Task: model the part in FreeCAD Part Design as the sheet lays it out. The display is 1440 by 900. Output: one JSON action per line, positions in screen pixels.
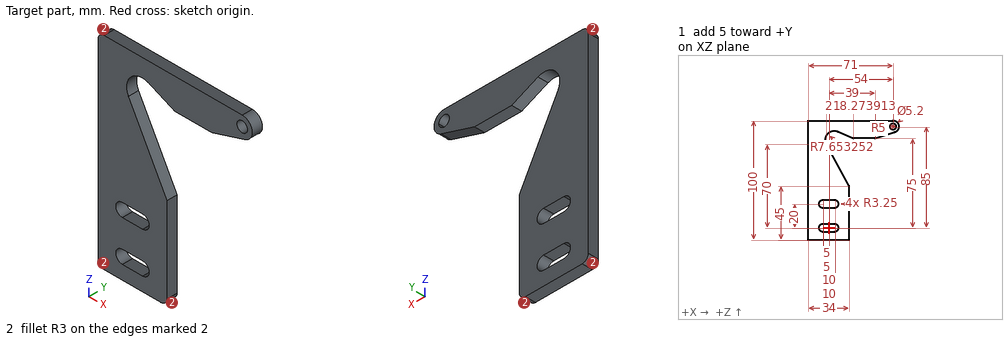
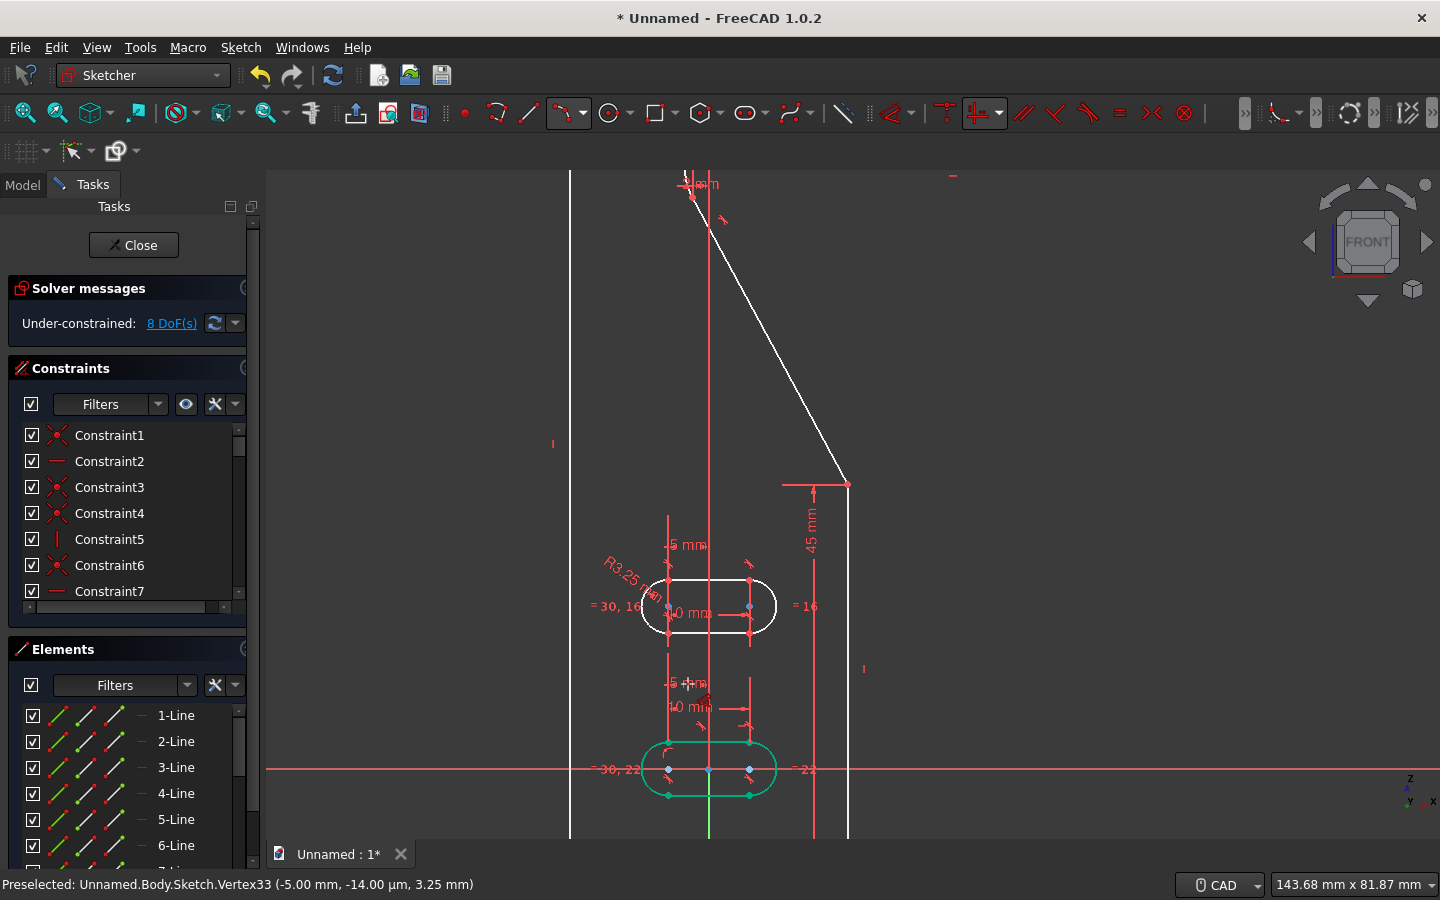
{"action": "scroll", "coordinate": [668, 580], "scroll_direction": "down", "scroll_amount": 3}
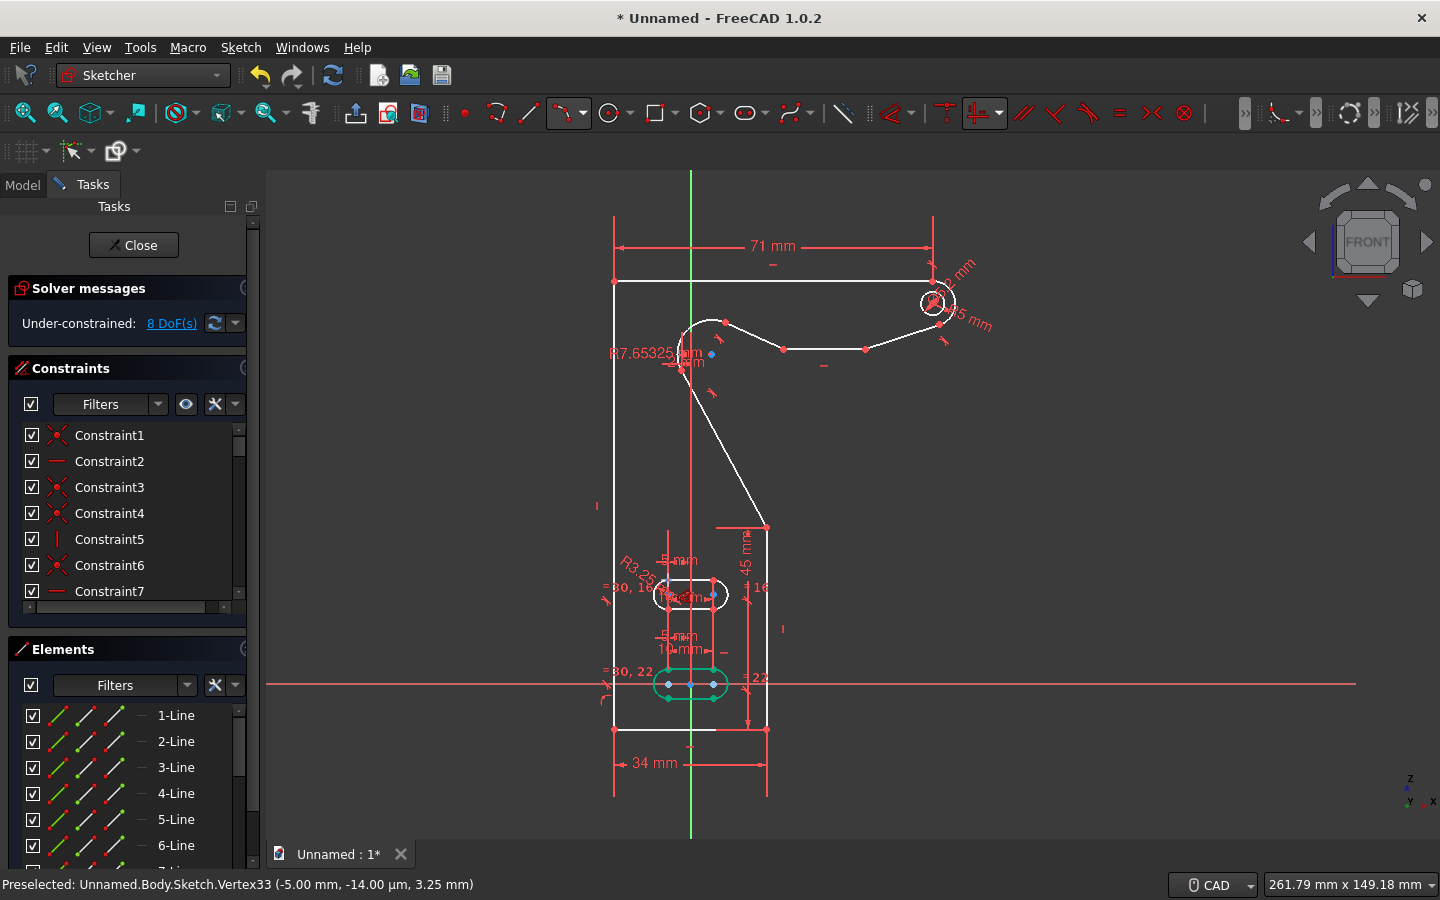
{"action": "left_click", "coordinate": [933, 304]}
{"action": "left_click", "coordinate": [812, 718]}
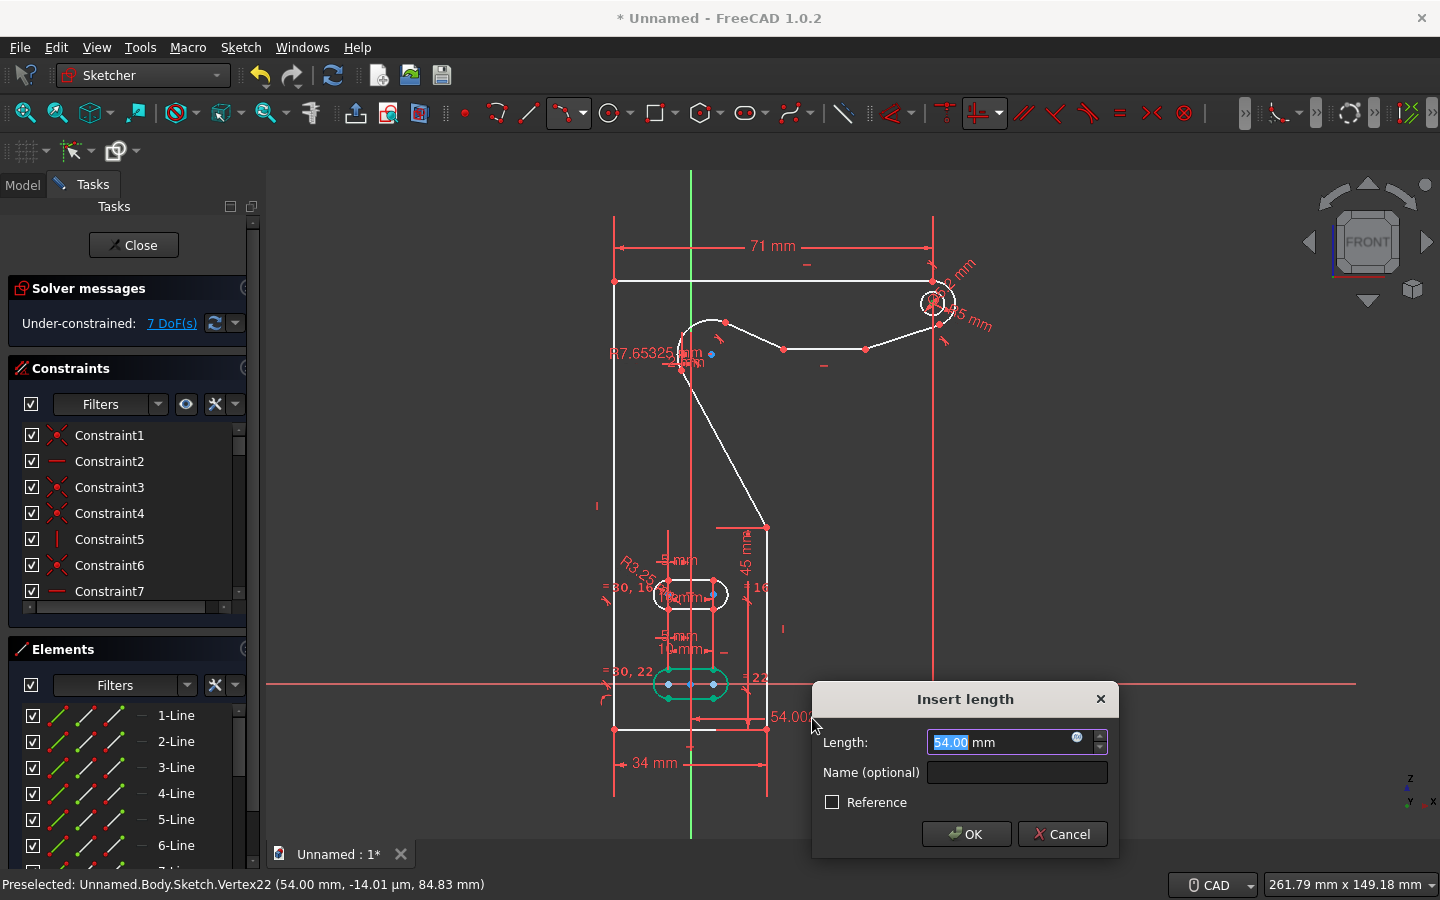
{"action": "type", "text": "54"}
{"action": "key", "text": "Return"}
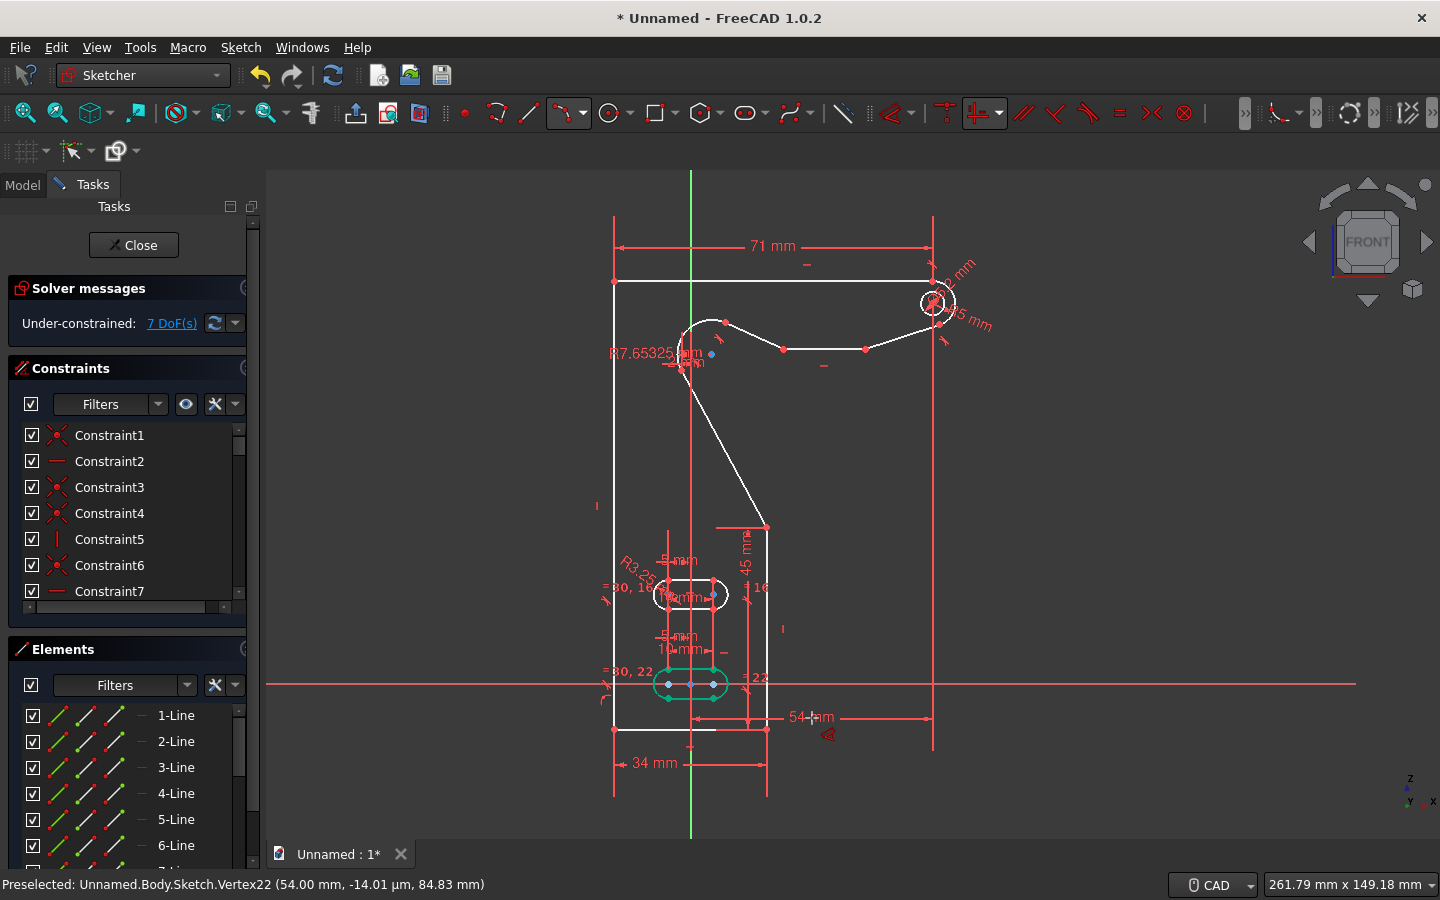
{"action": "left_click", "coordinate": [933, 304]}
{"action": "left_click", "coordinate": [967, 494]}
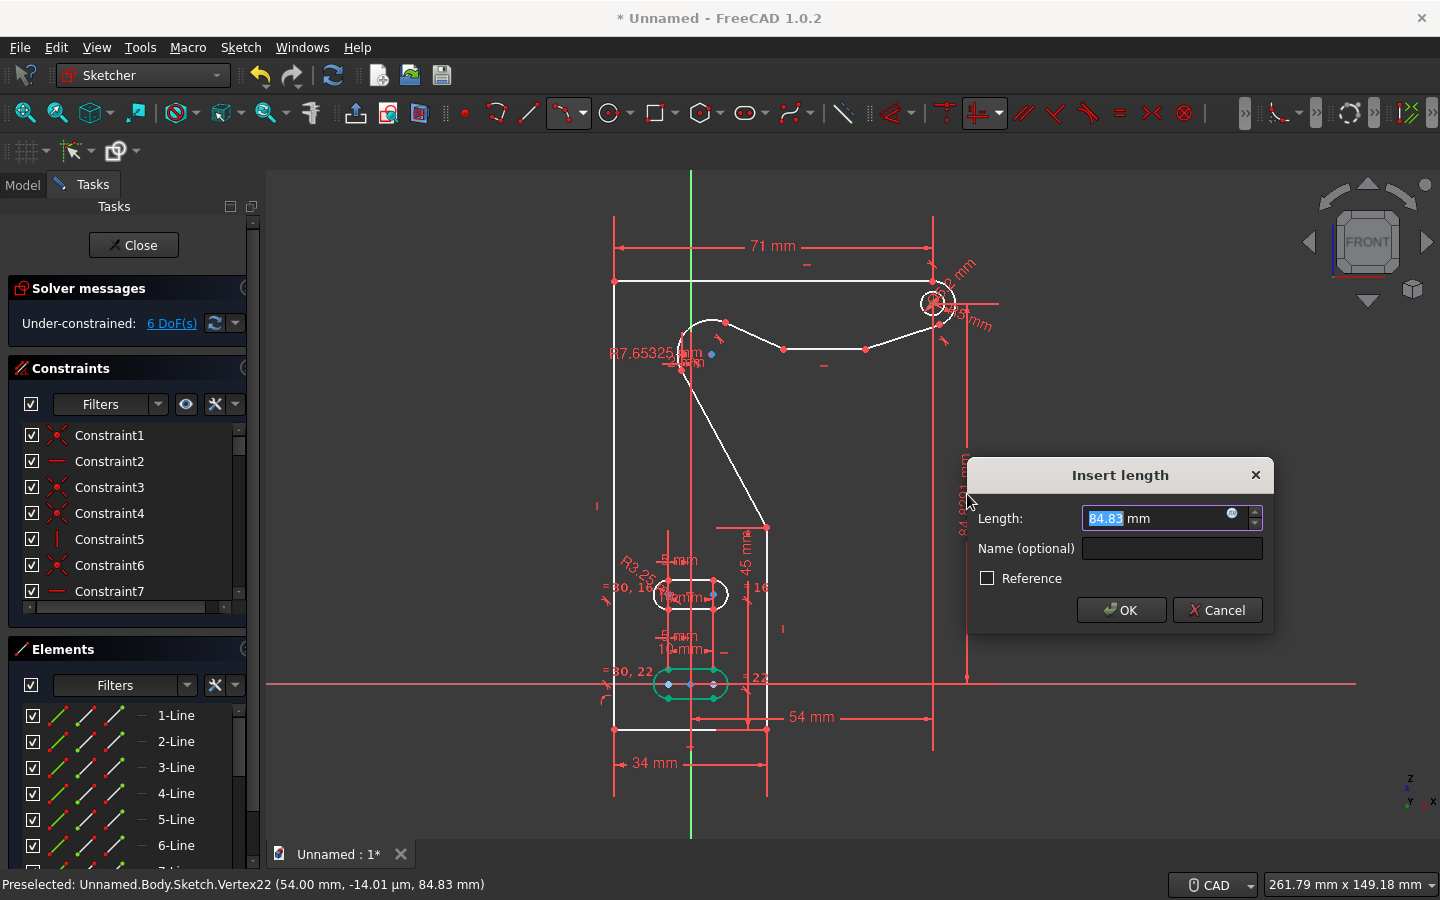
{"action": "type", "text": "85"}
{"action": "key", "text": "Return"}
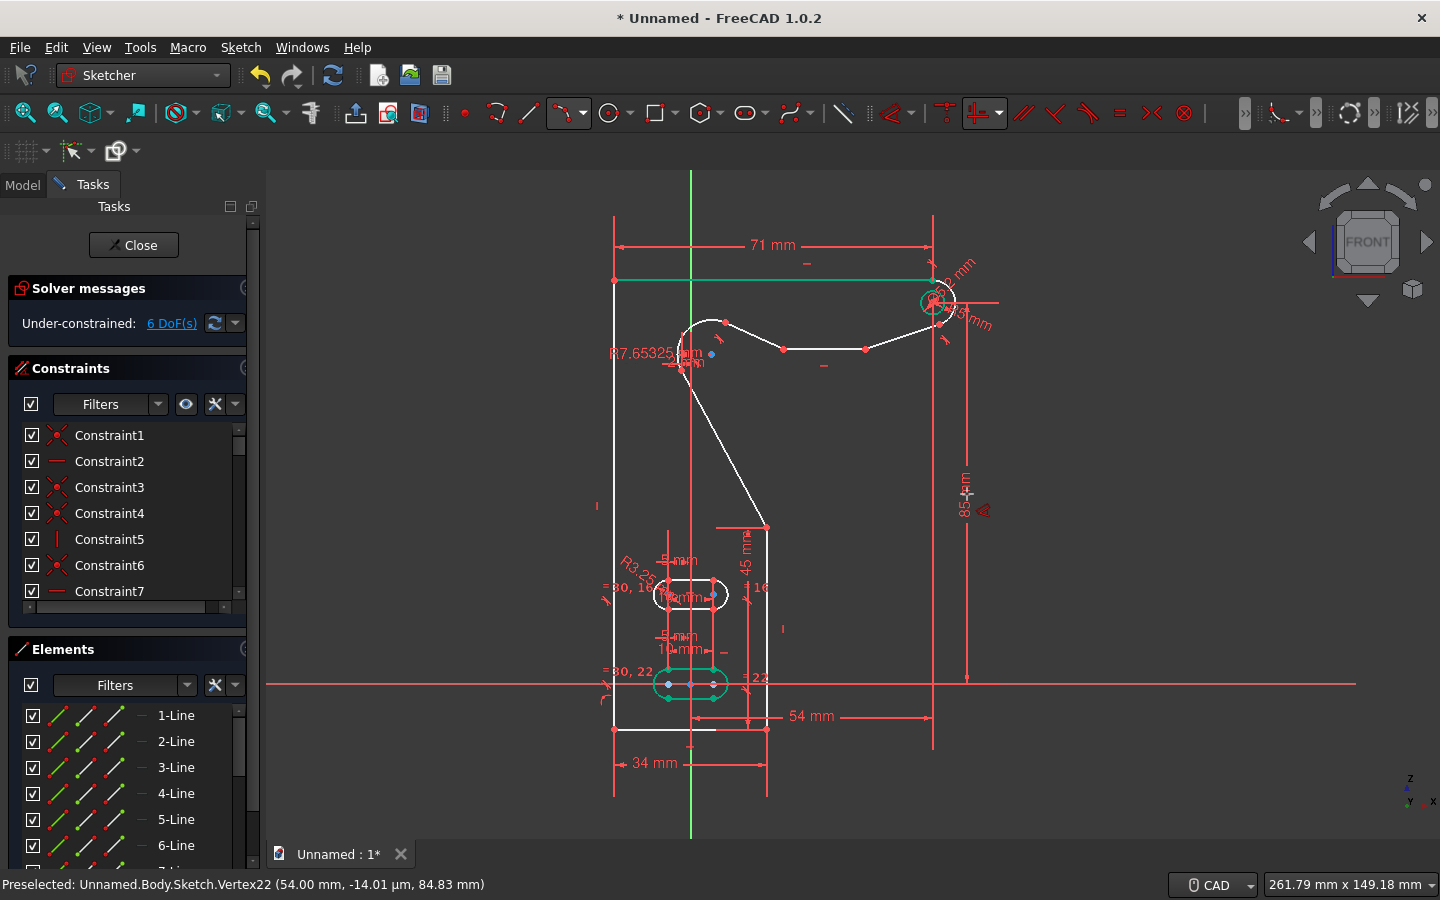
{"action": "left_click", "coordinate": [614, 595]}
{"action": "left_click", "coordinate": [580, 505]}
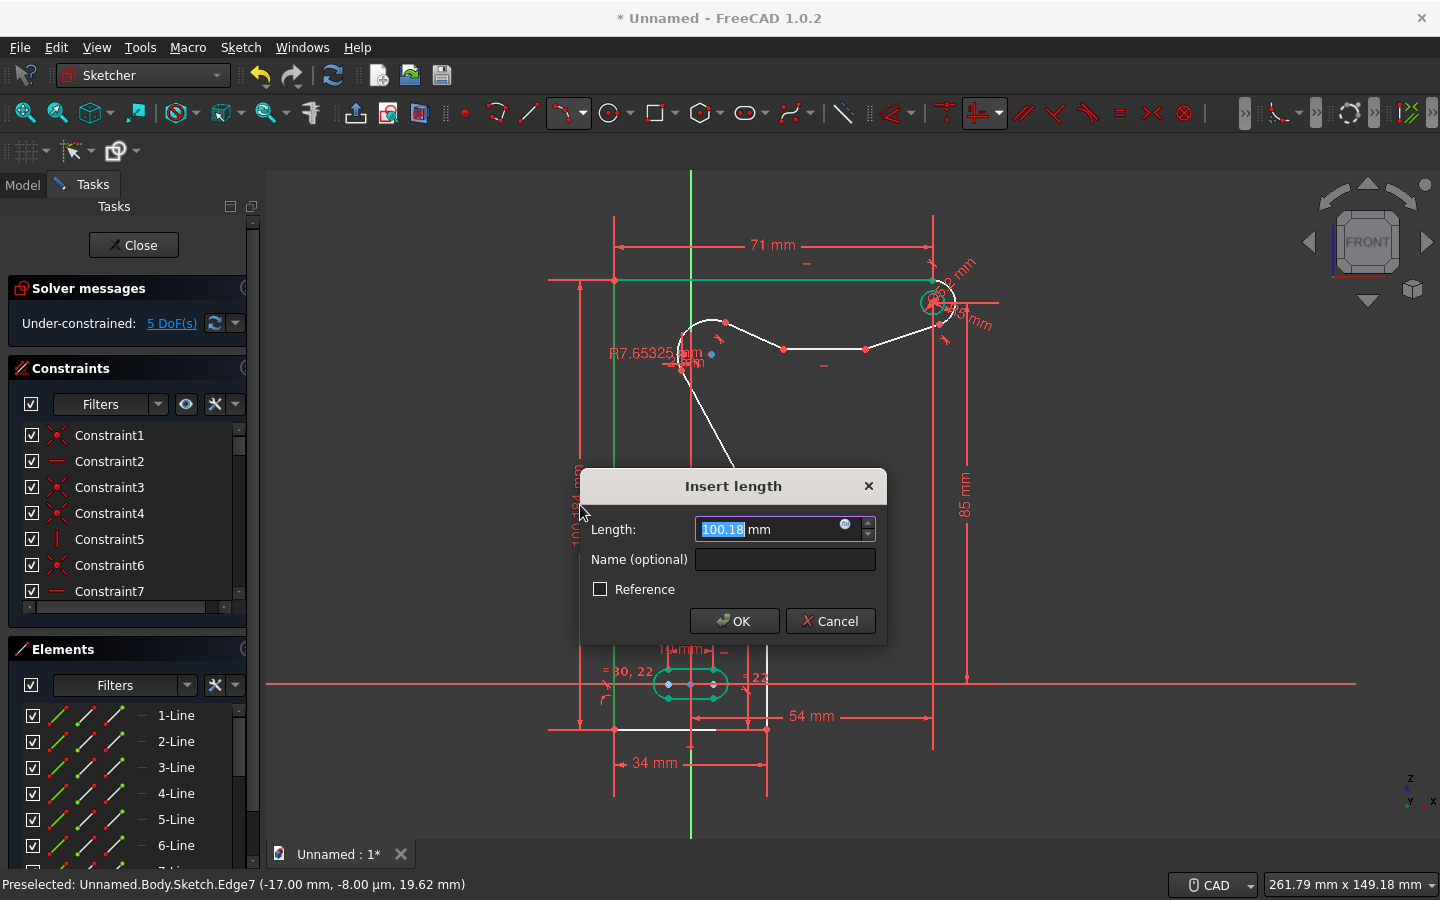
{"action": "type", "text": "100"}
{"action": "key", "text": "Return"}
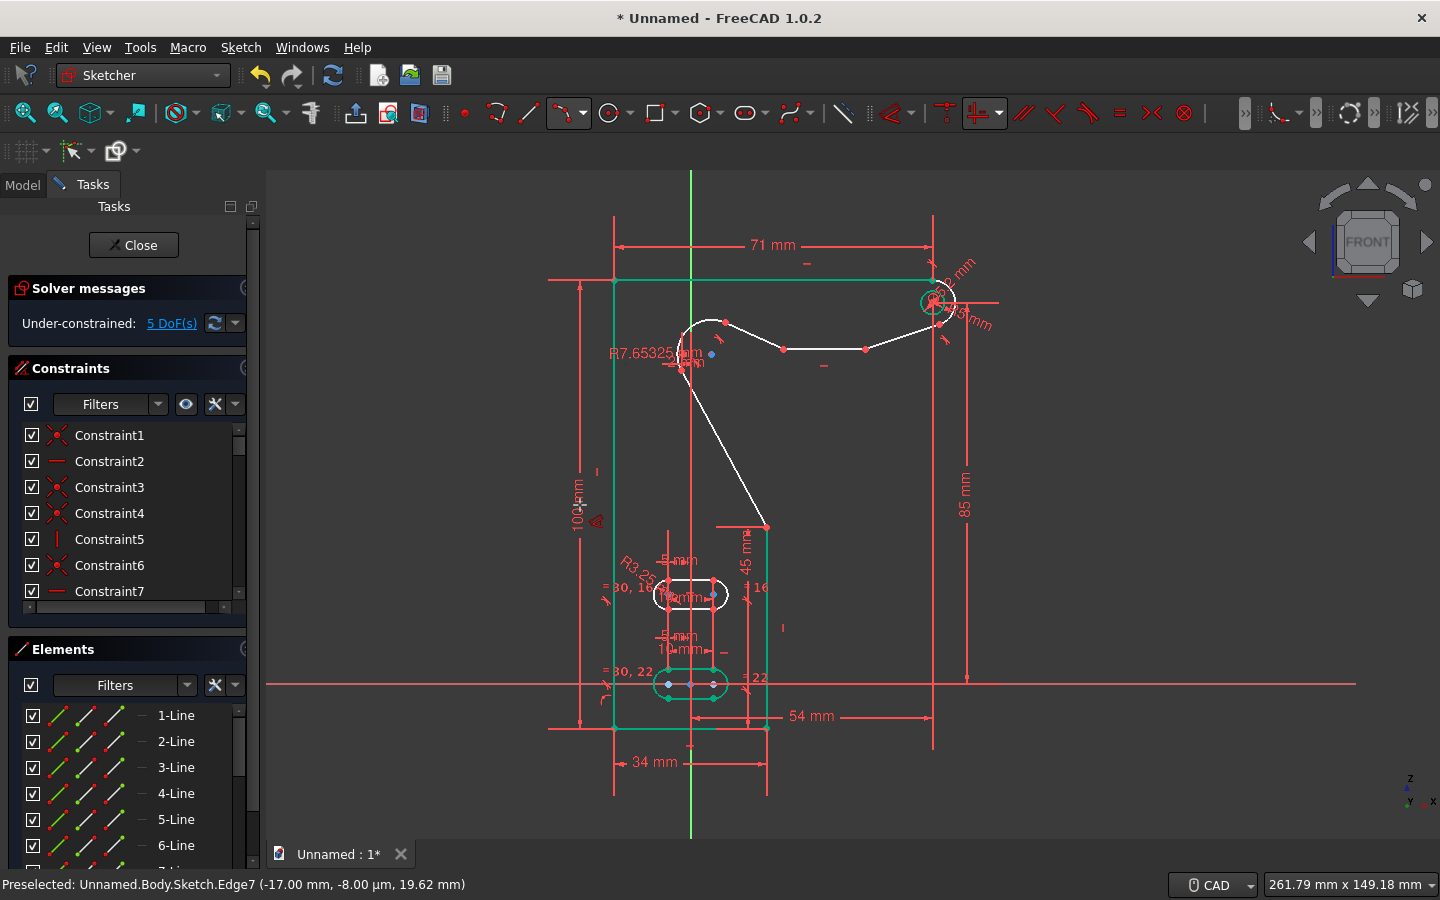
{"action": "left_click", "coordinate": [865, 349]}
{"action": "left_click", "coordinate": [778, 315]}